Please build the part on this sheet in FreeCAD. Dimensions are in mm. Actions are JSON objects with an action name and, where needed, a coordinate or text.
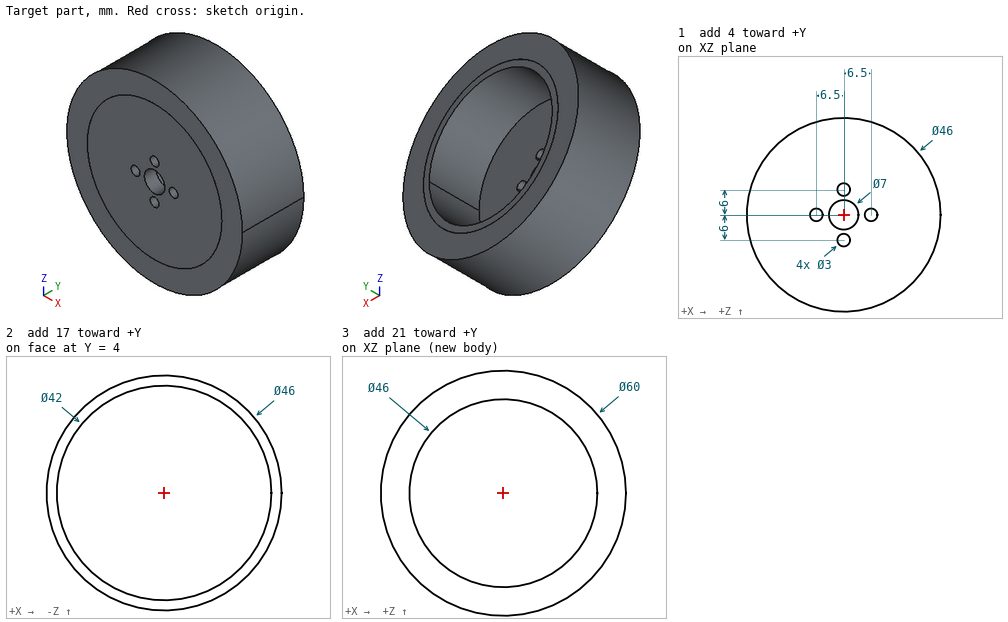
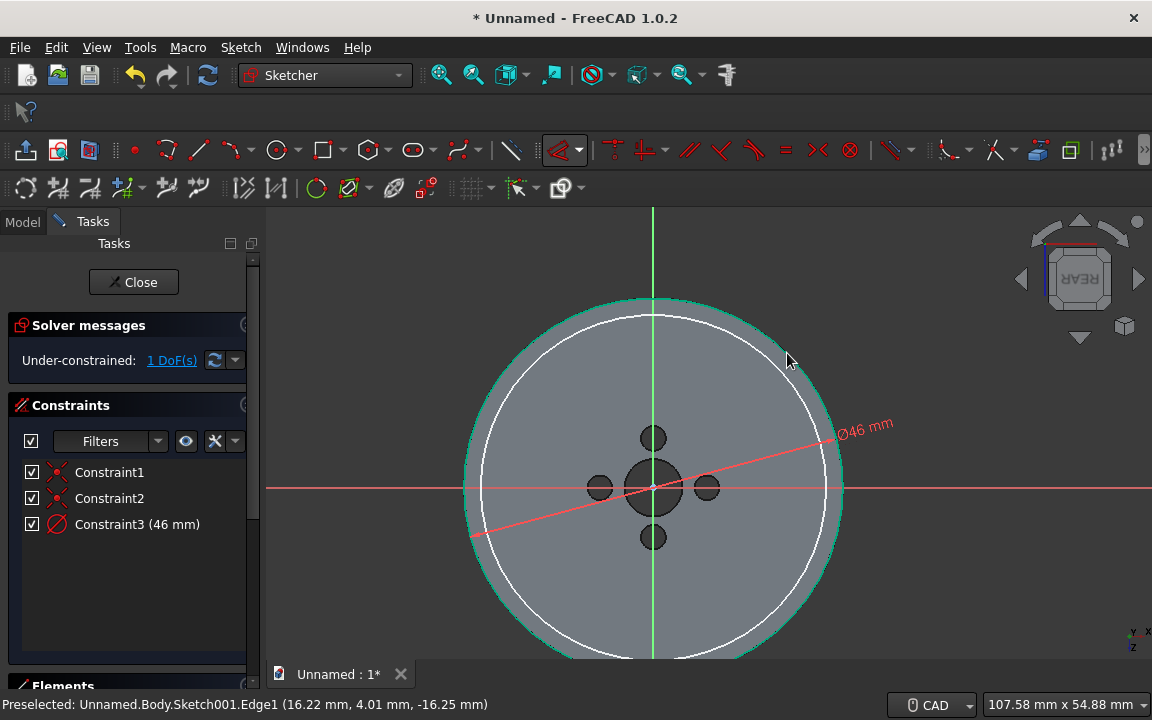
{"action": "left_click", "coordinate": [775, 365]}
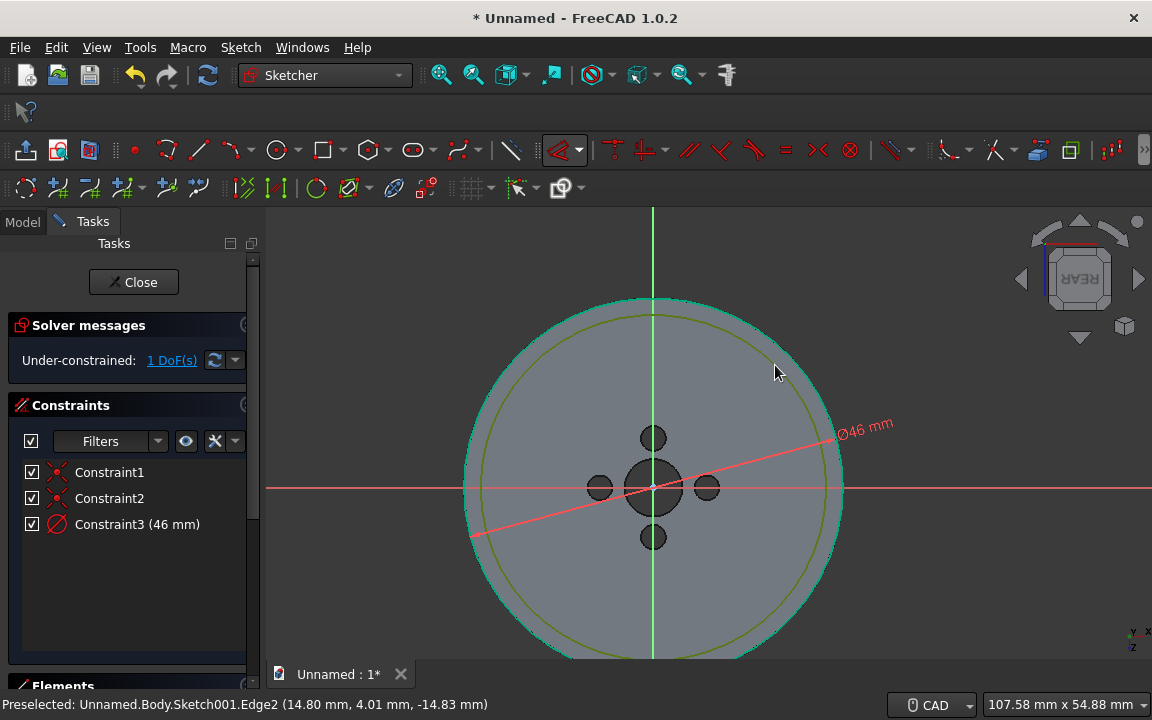
{"action": "left_click", "coordinate": [582, 150]}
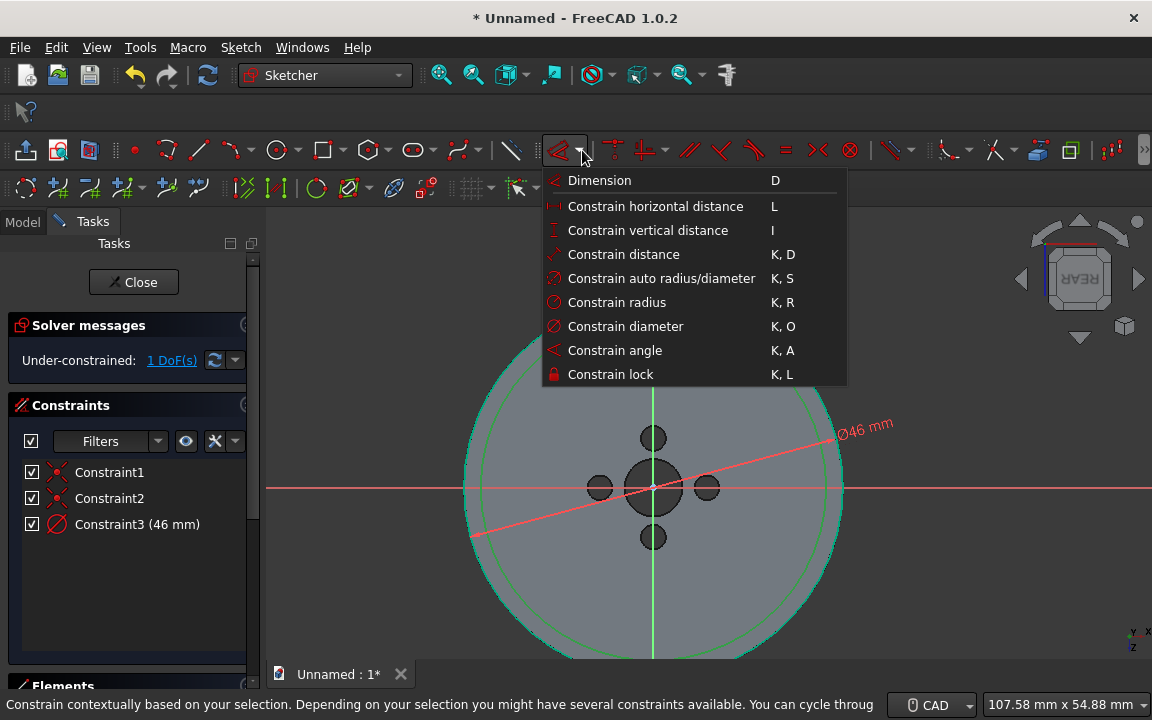
{"action": "left_click", "coordinate": [695, 326]}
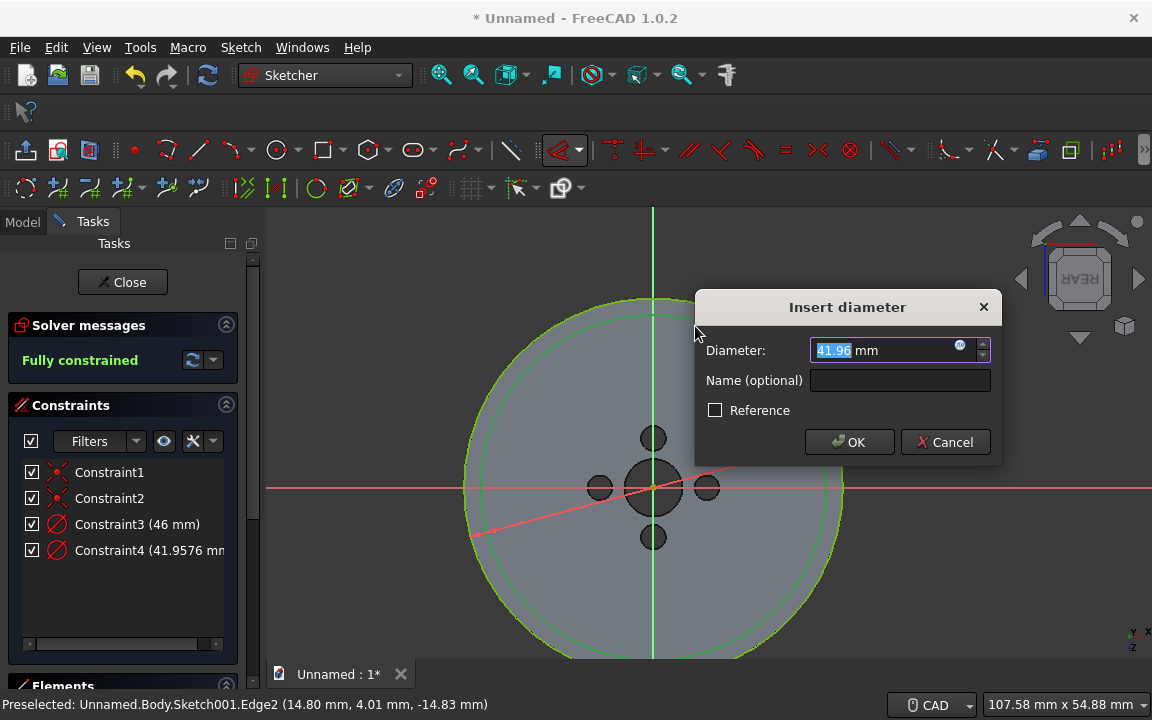
{"action": "type", "text": "42"}
{"action": "key", "text": "Return"}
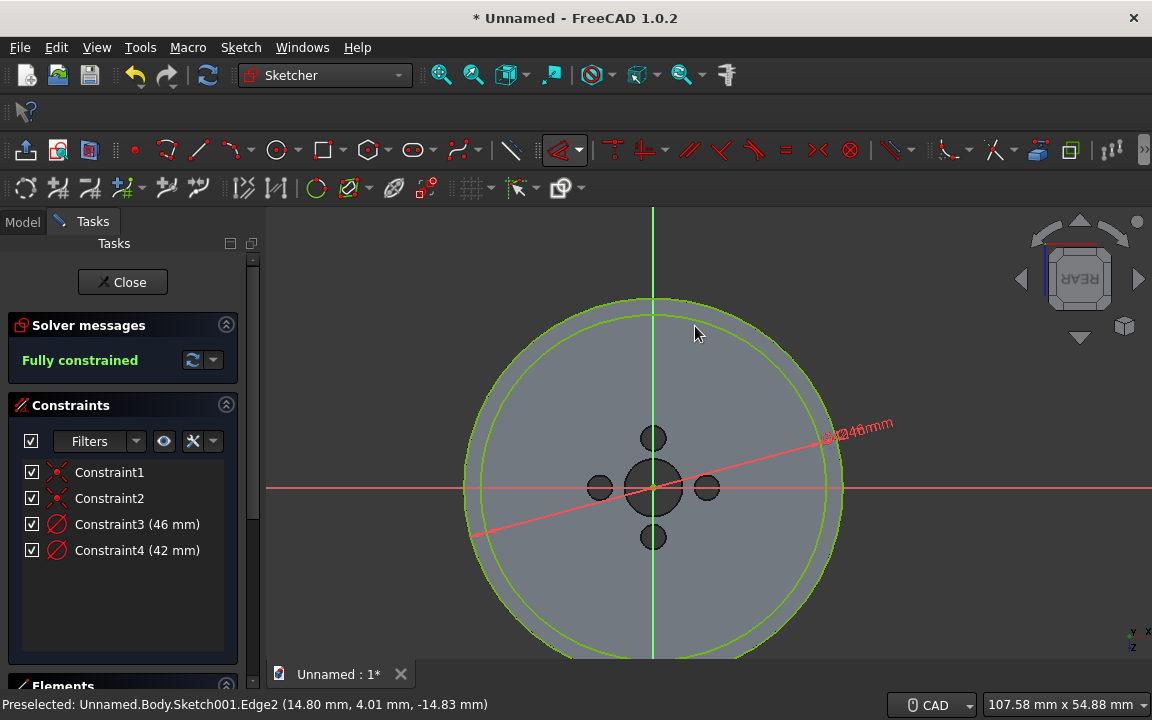
{"action": "left_click", "coordinate": [123, 282]}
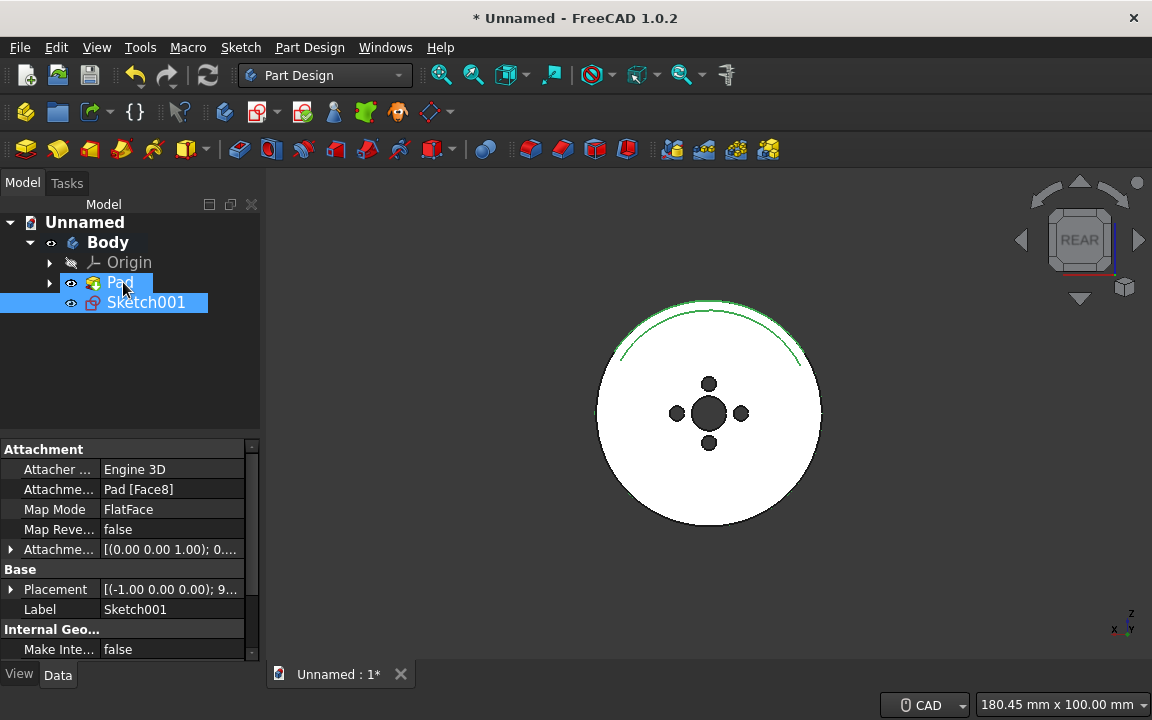
{"action": "left_click", "coordinate": [26, 150]}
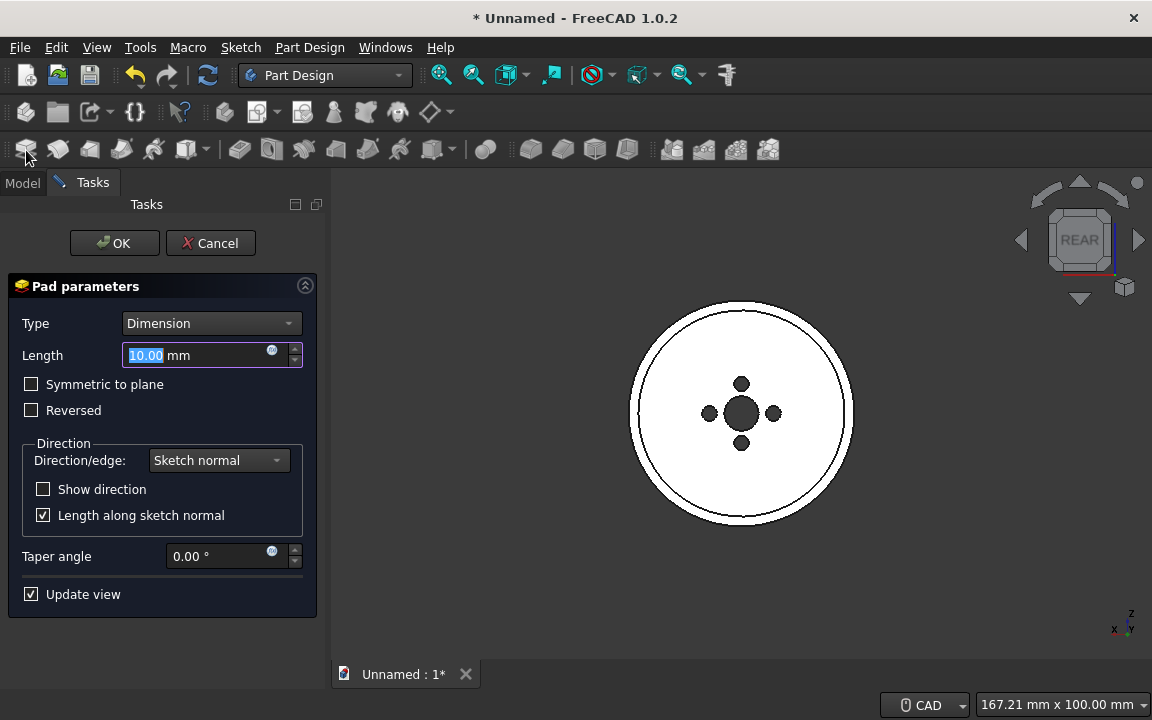
{"action": "type", "text": "17"}
{"action": "key", "text": "Tab"}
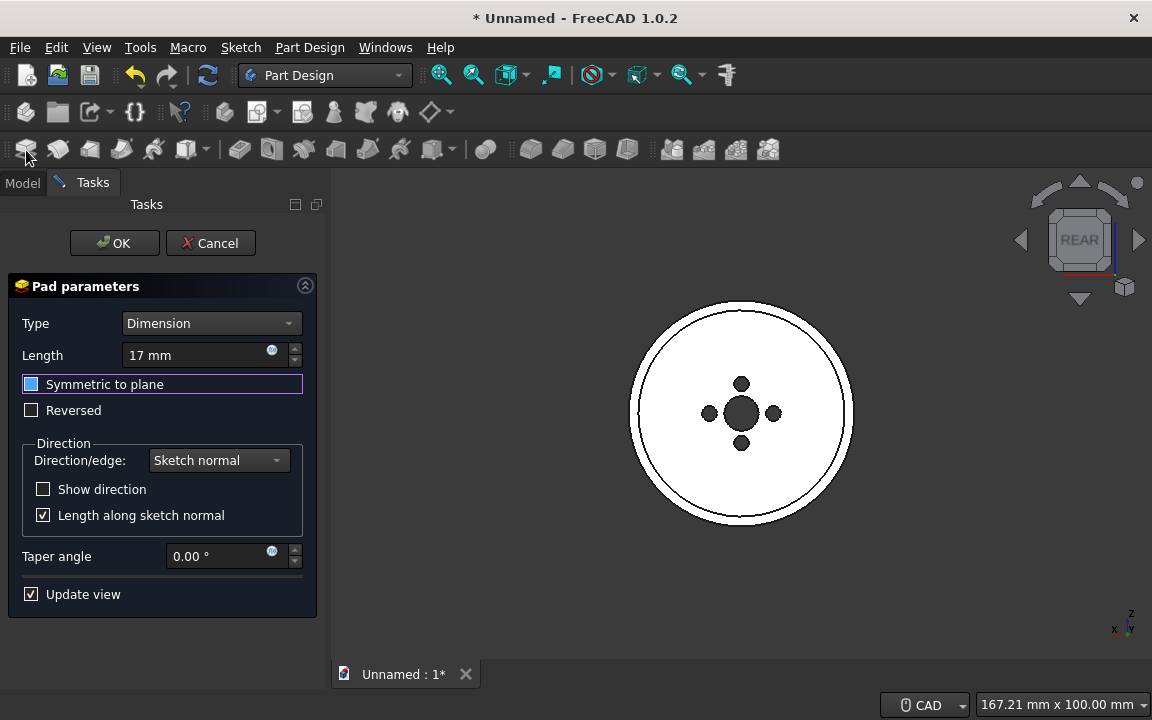
{"action": "left_click", "coordinate": [115, 243]}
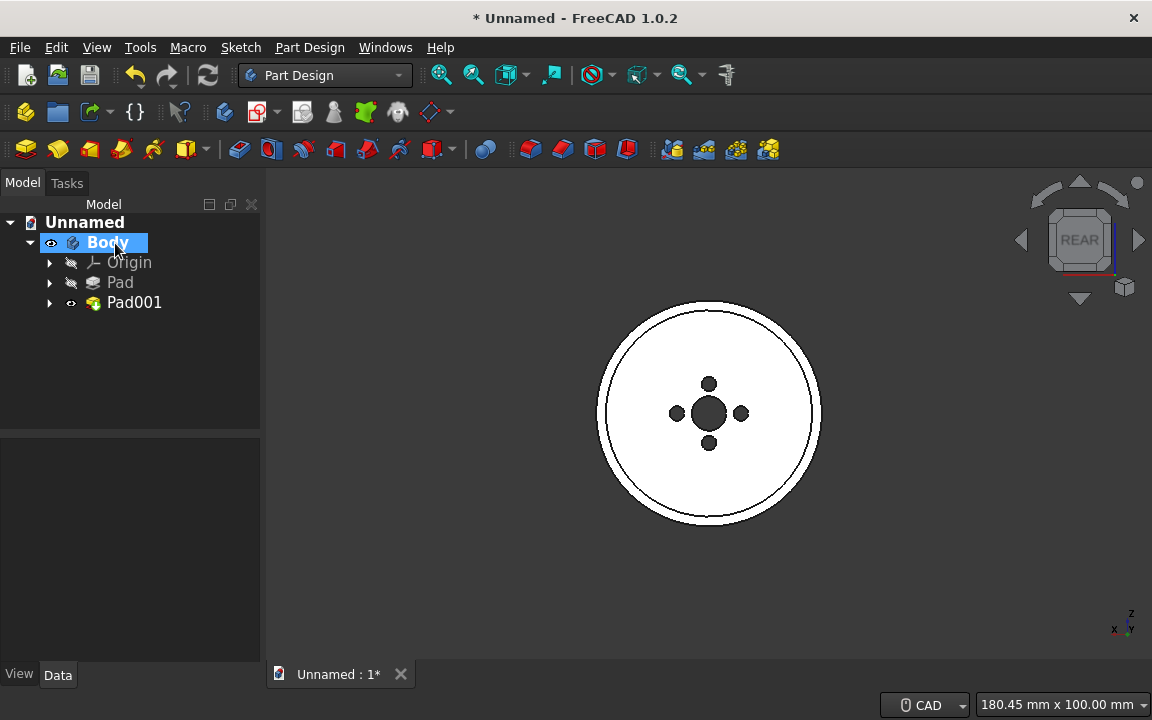
{"action": "left_click", "coordinate": [226, 112]}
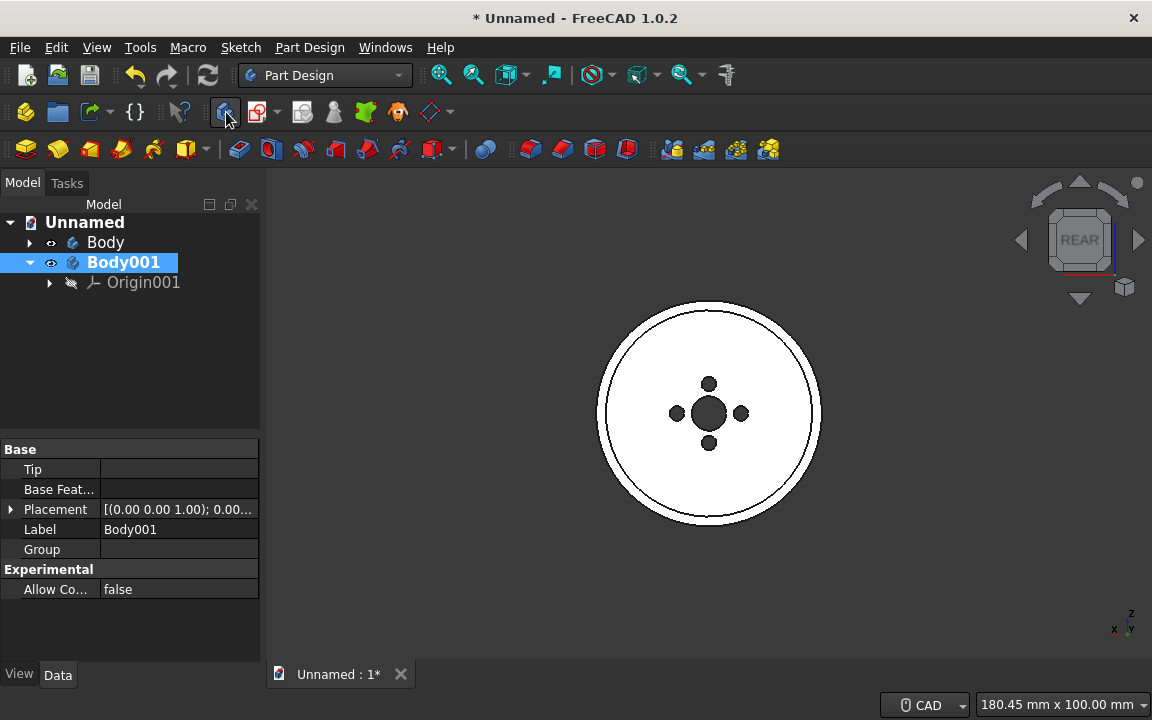
{"action": "left_click", "coordinate": [306, 619]}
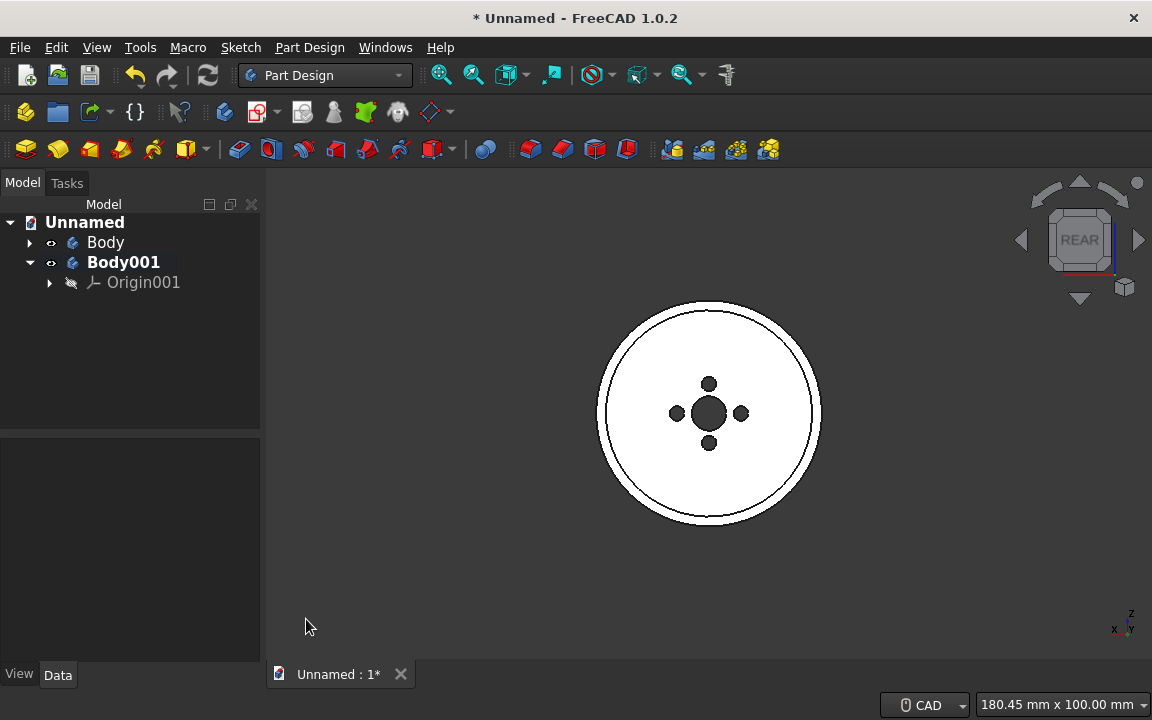
{"action": "left_click", "coordinate": [258, 112]}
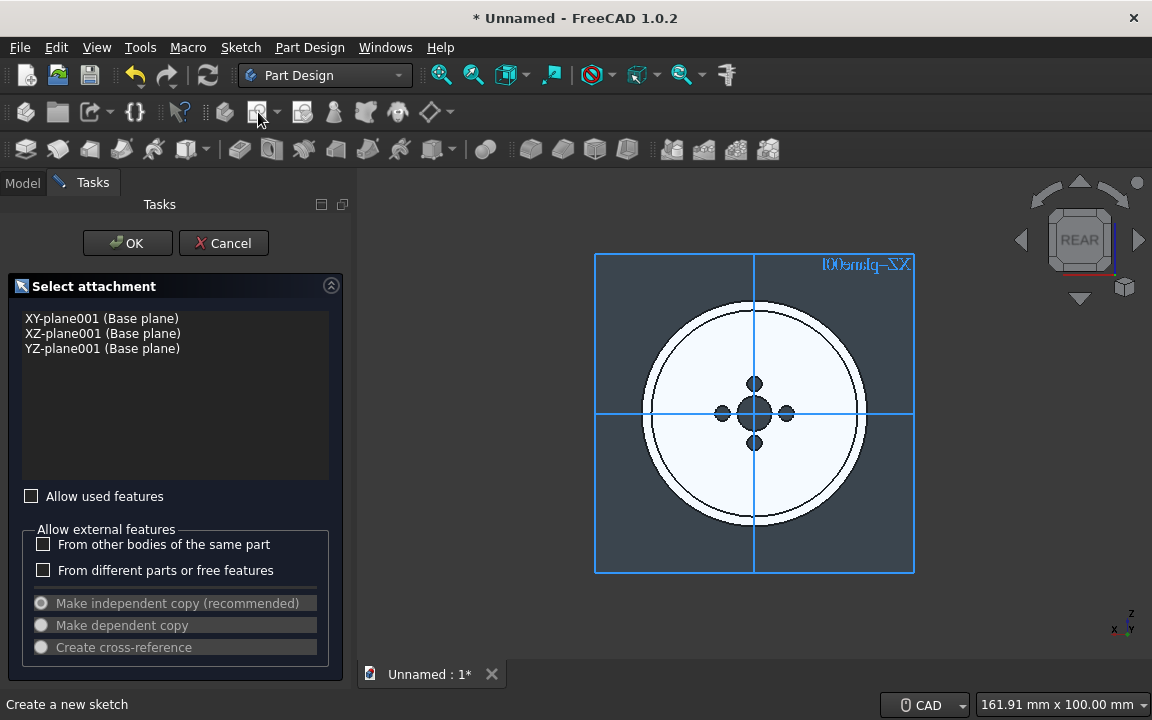
{"action": "left_click", "coordinate": [82, 334]}